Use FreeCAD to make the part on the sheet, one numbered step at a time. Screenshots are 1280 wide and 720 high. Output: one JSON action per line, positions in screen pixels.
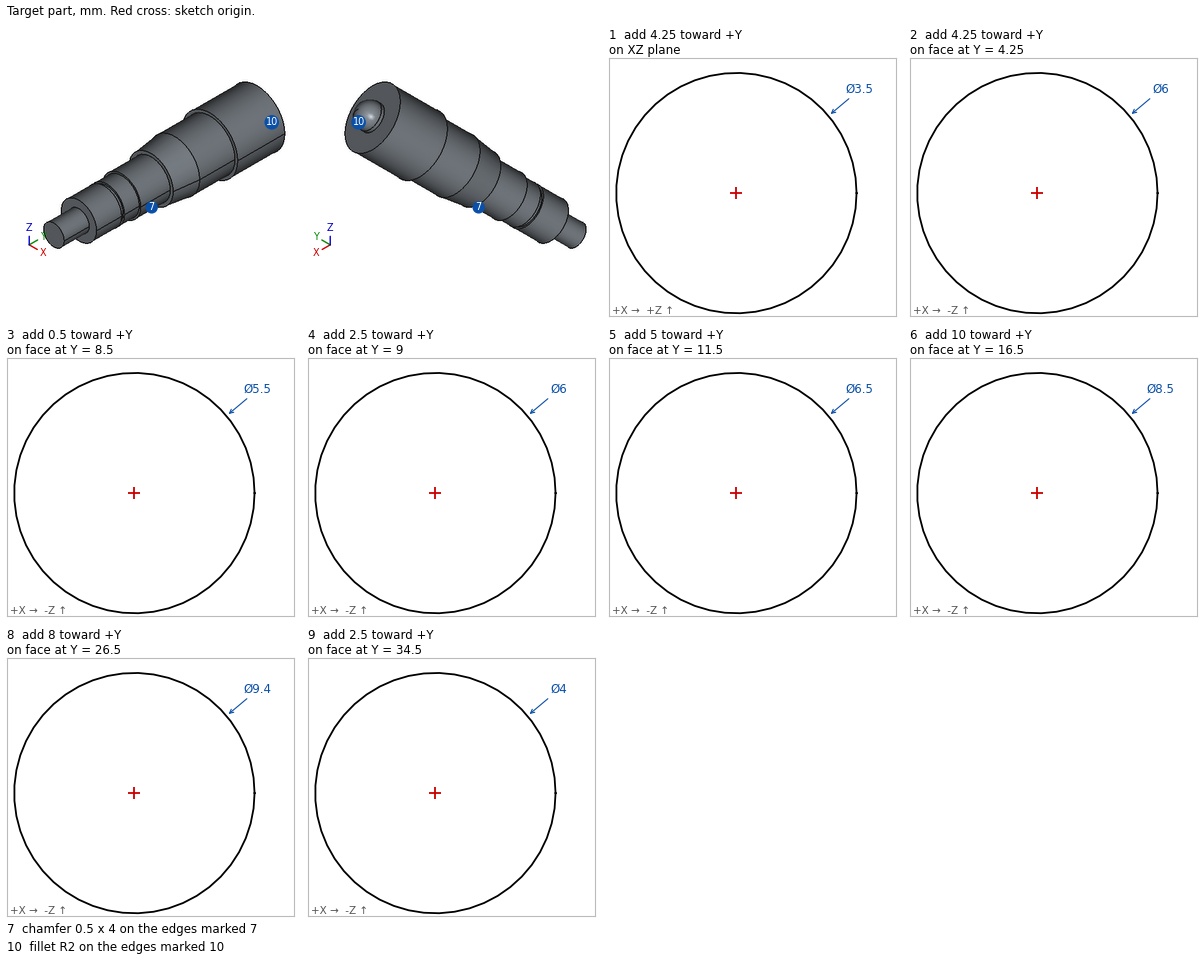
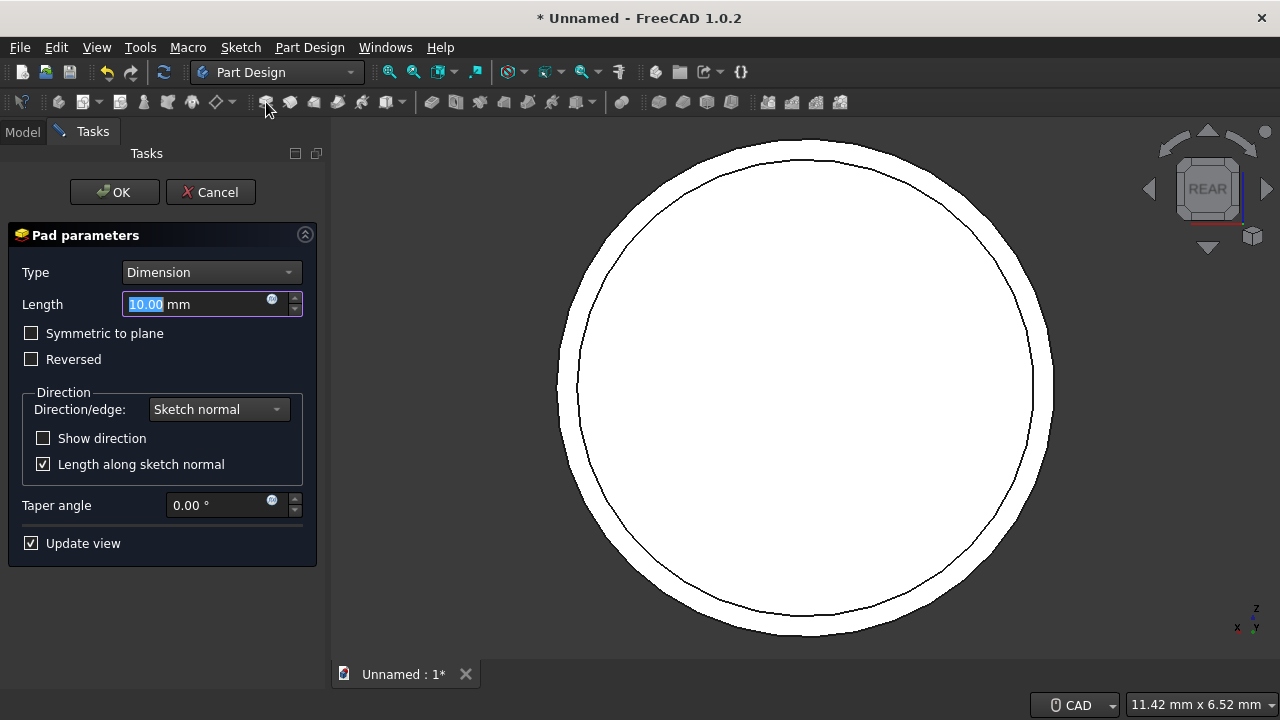
{"action": "type", "text": "0.5"}
{"action": "key", "text": "Tab"}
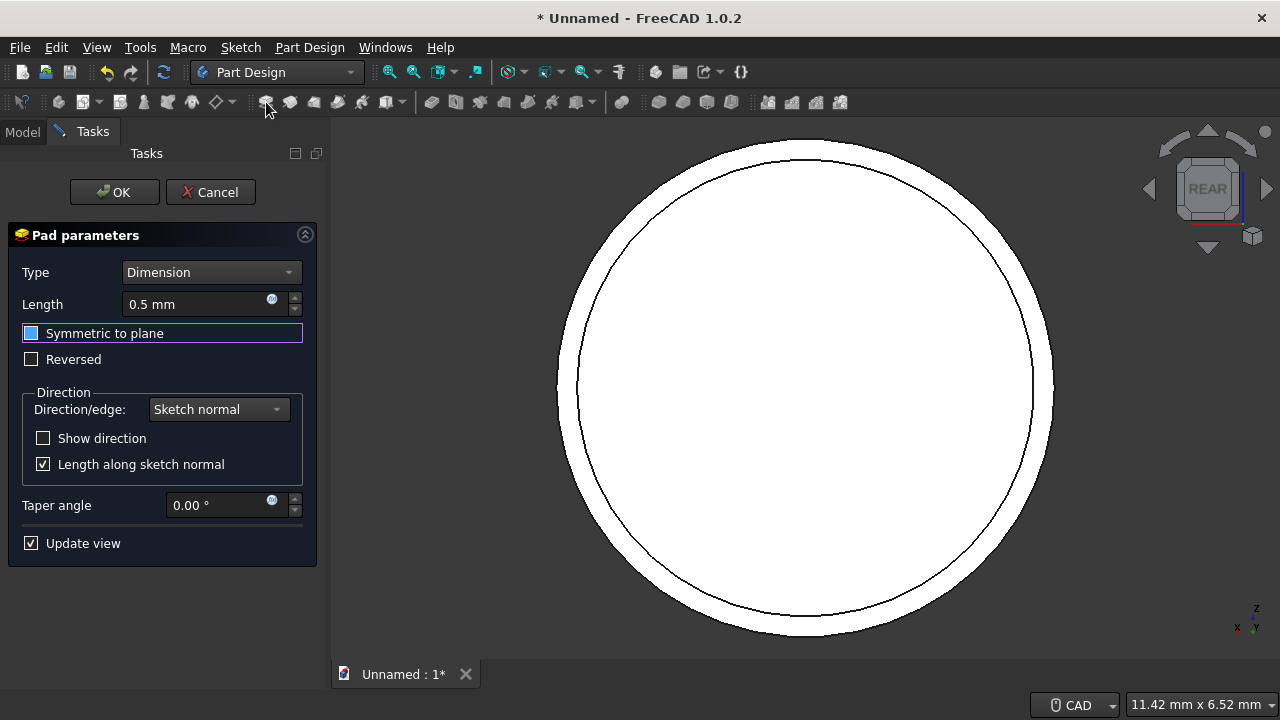
{"action": "left_click", "coordinate": [115, 192]}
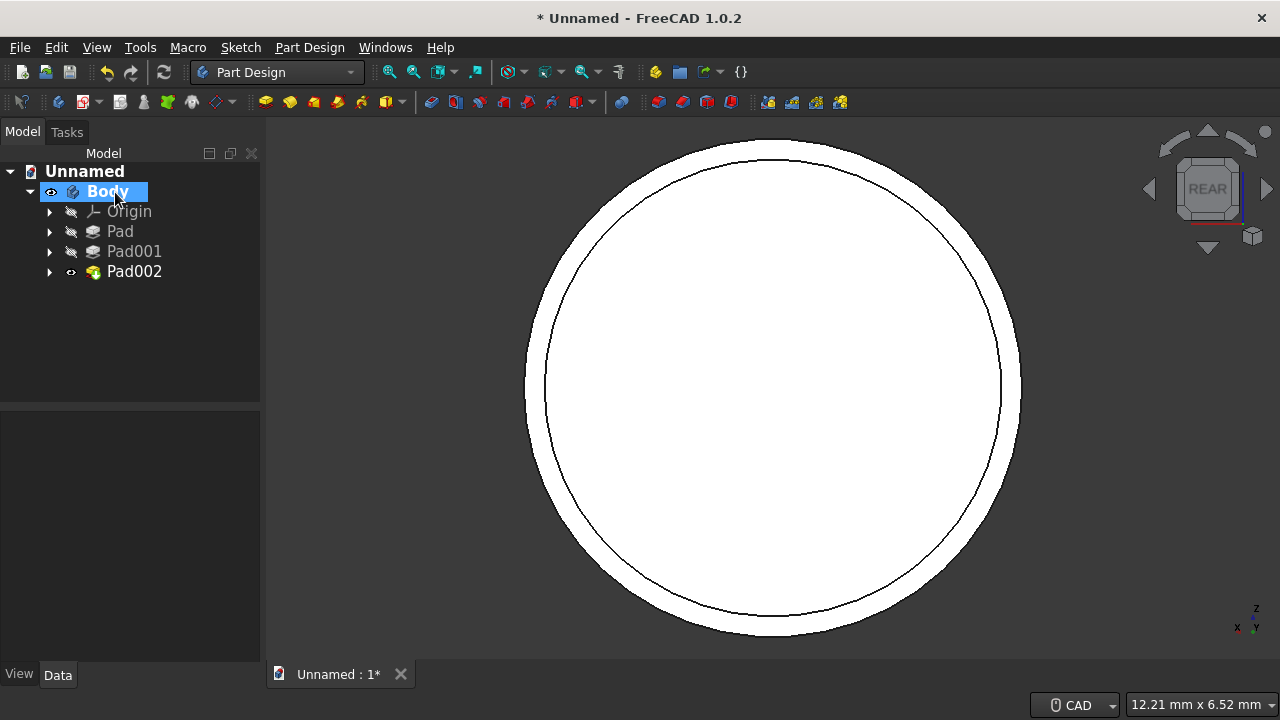
{"action": "left_click", "coordinate": [773, 387]}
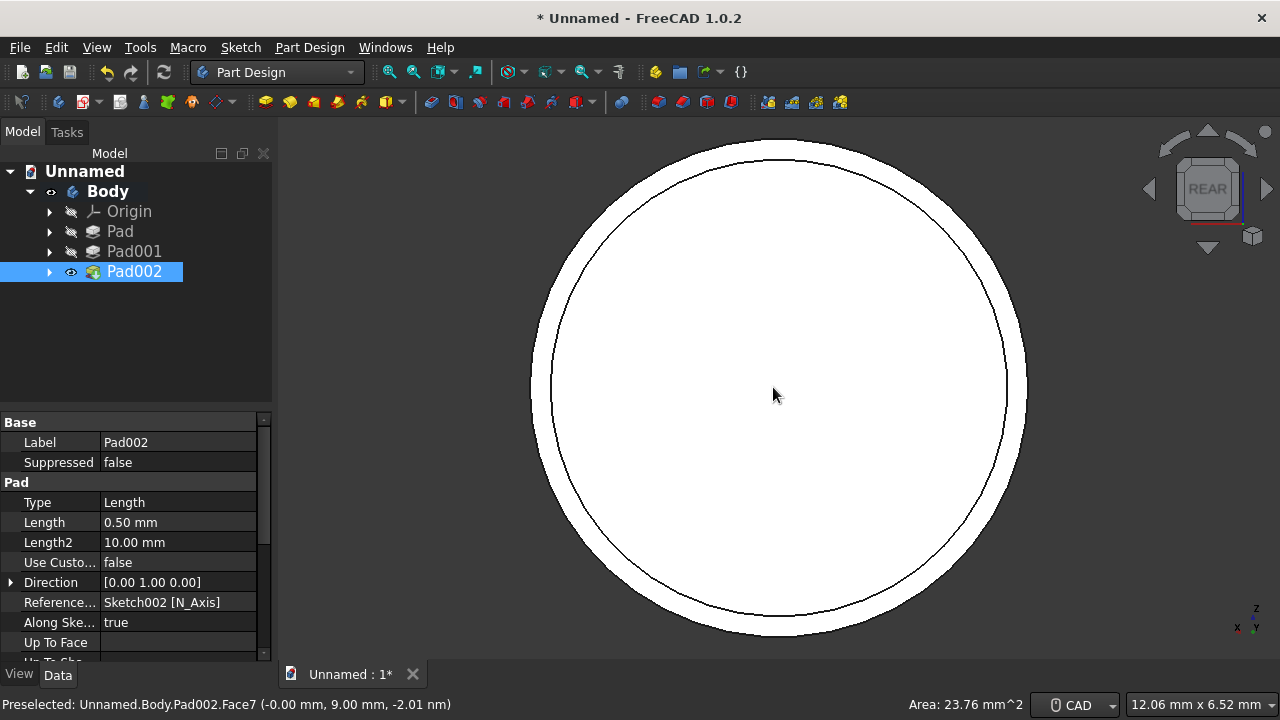
{"action": "left_click", "coordinate": [84, 102]}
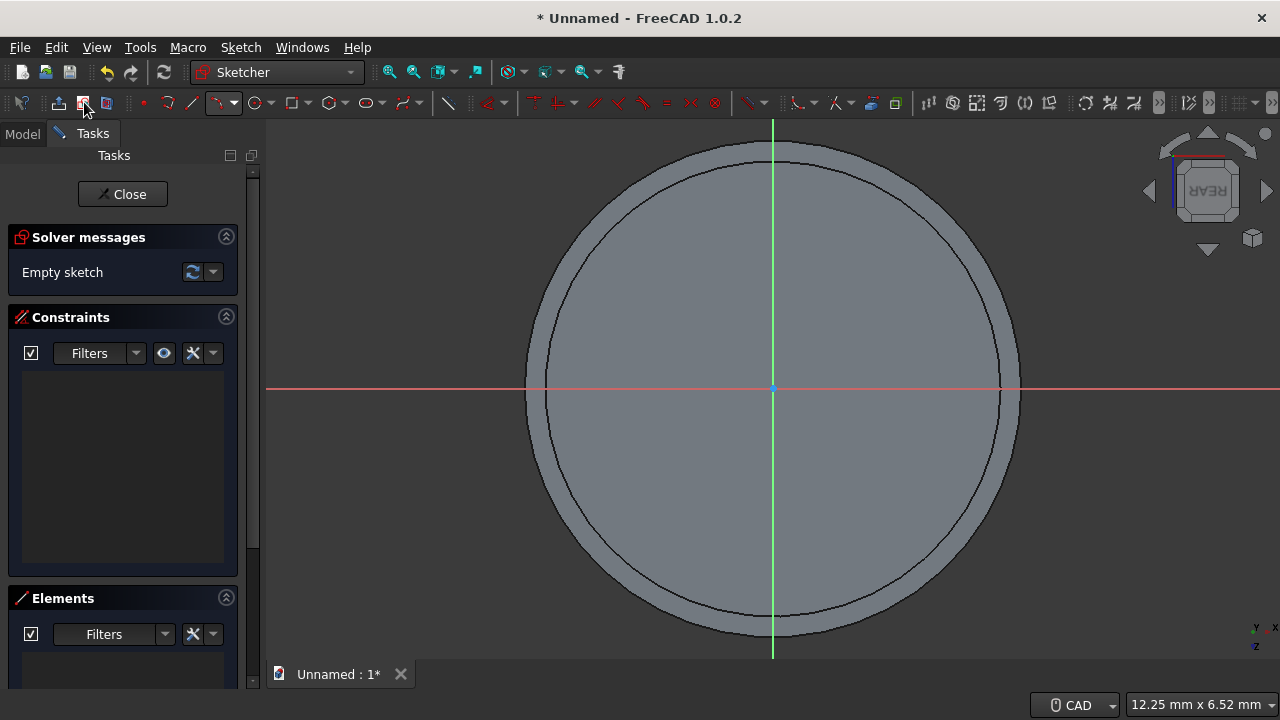
{"action": "scroll", "coordinate": [565, 389], "scroll_direction": "down", "scroll_amount": 2}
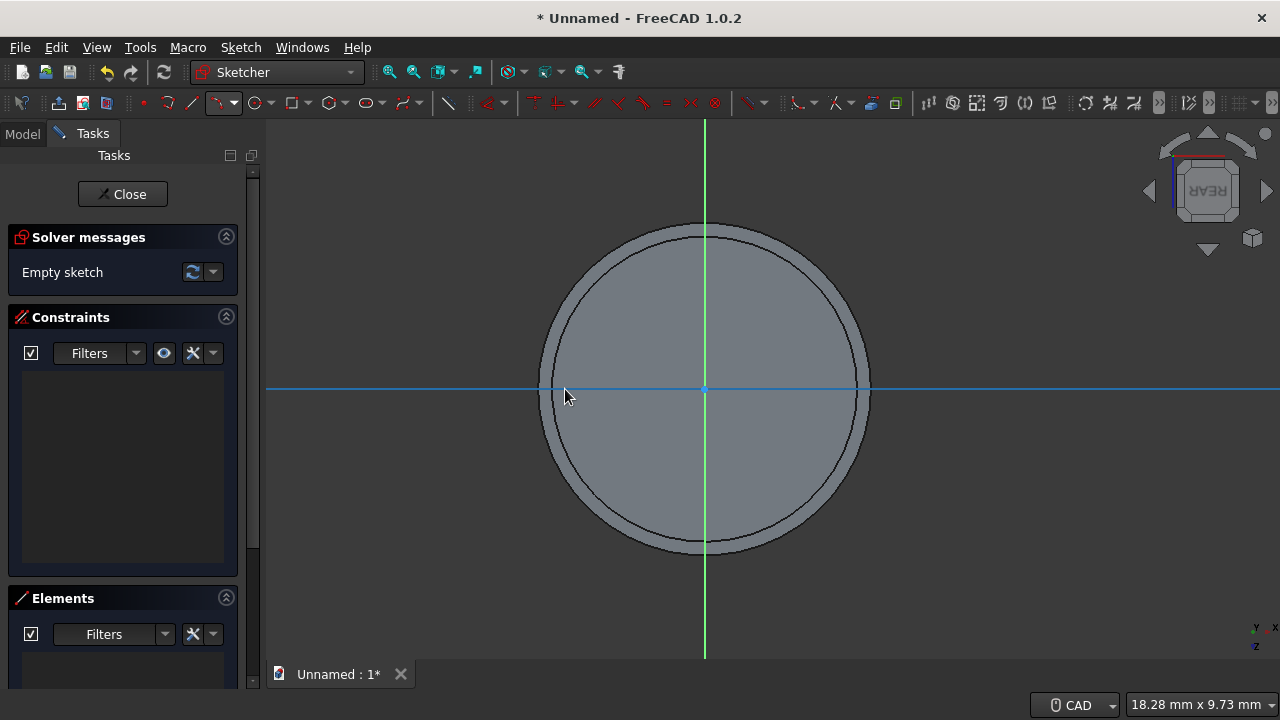
{"action": "key", "text": "g c"}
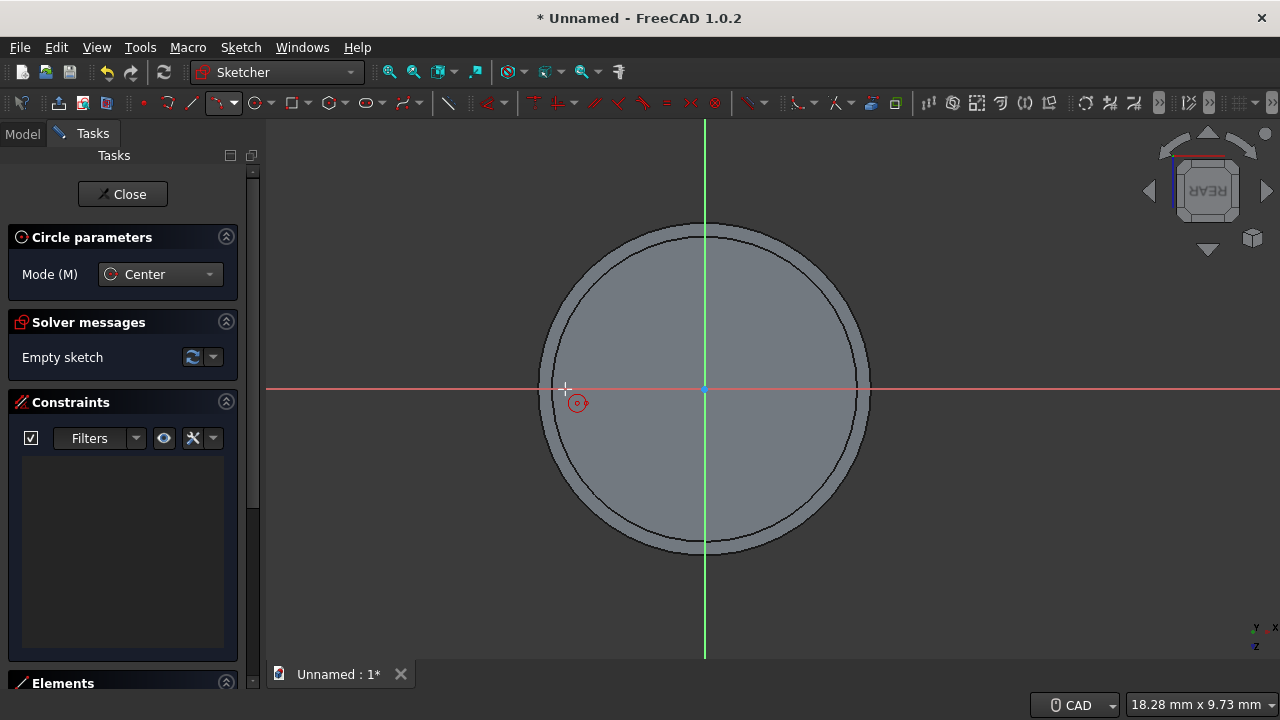
{"action": "left_click", "coordinate": [705, 389]}
{"action": "mouse_move", "coordinate": [822, 271]}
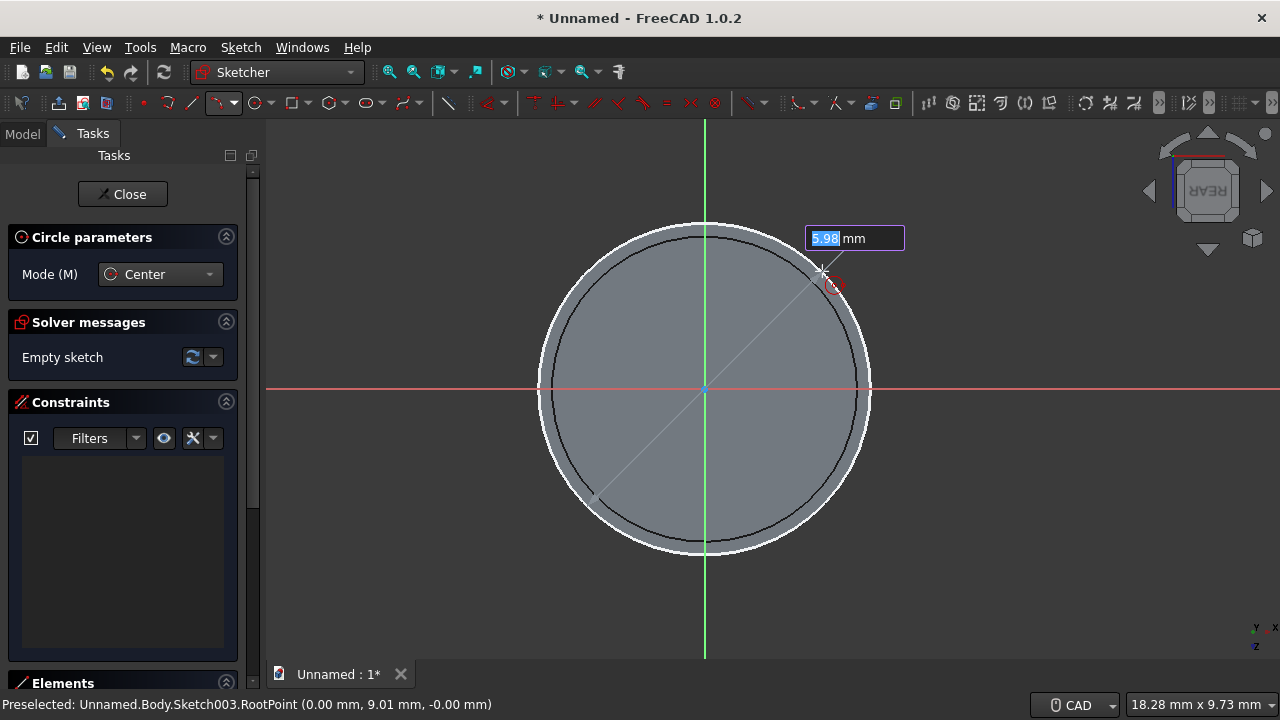
{"action": "type", "text": "6"}
{"action": "key", "text": "Return"}
{"action": "key", "text": "Escape"}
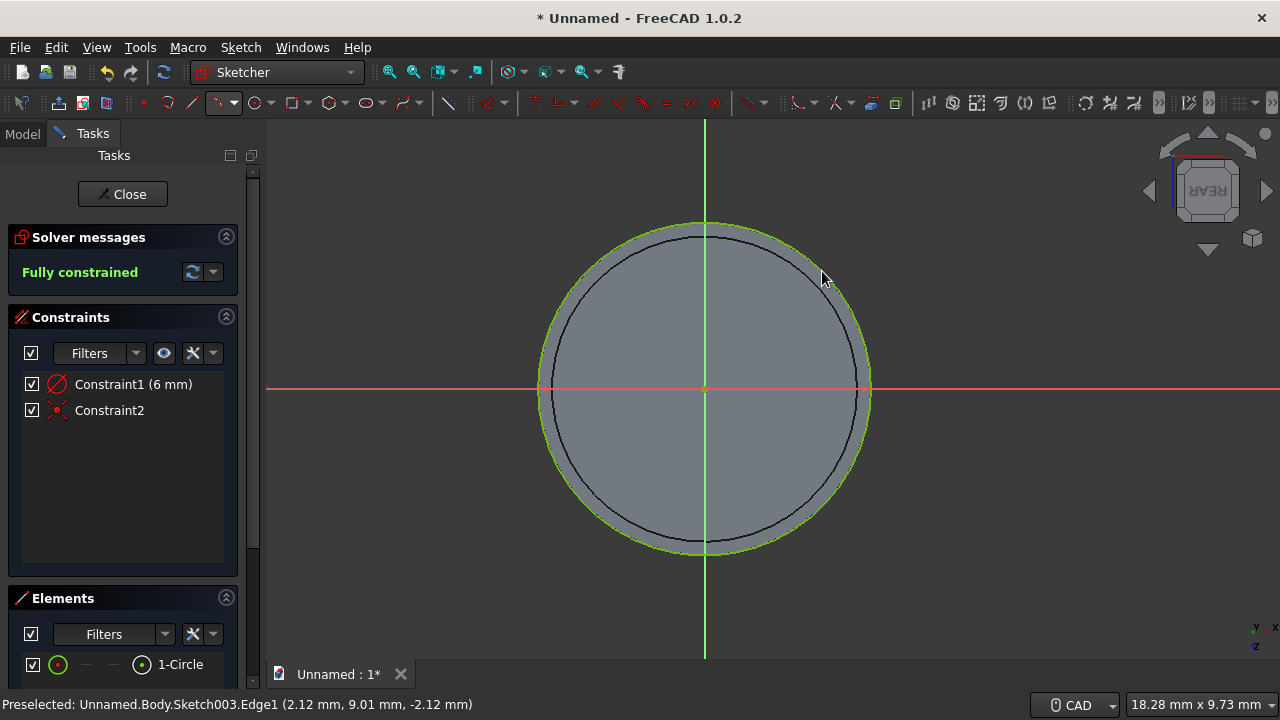
{"action": "left_click", "coordinate": [123, 194]}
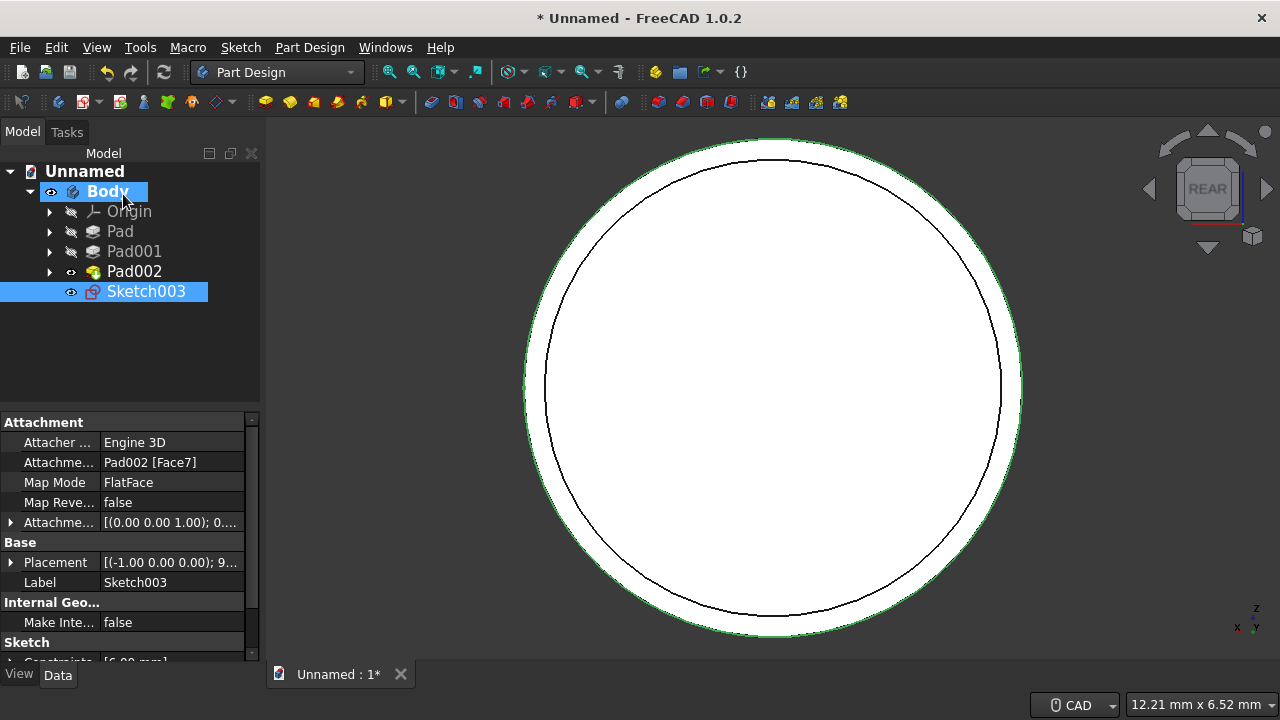
{"action": "left_click", "coordinate": [266, 102]}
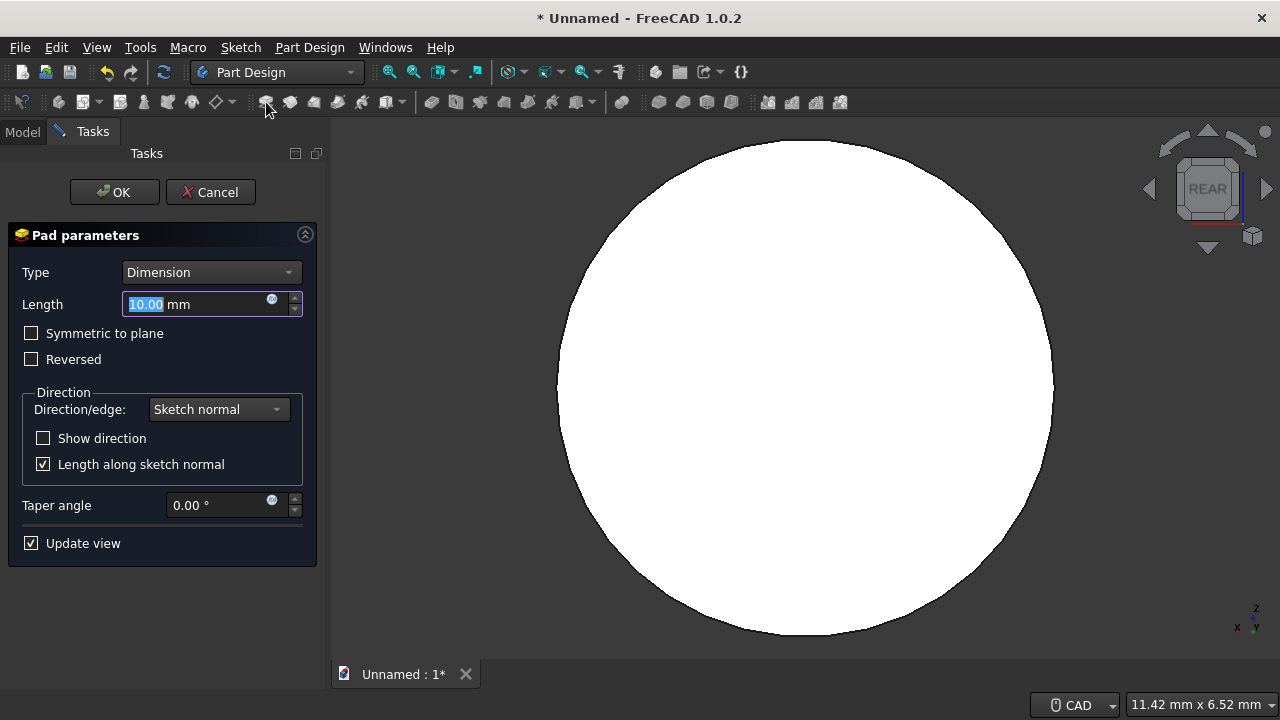
{"action": "type", "text": "2.5"}
{"action": "key", "text": "Tab"}